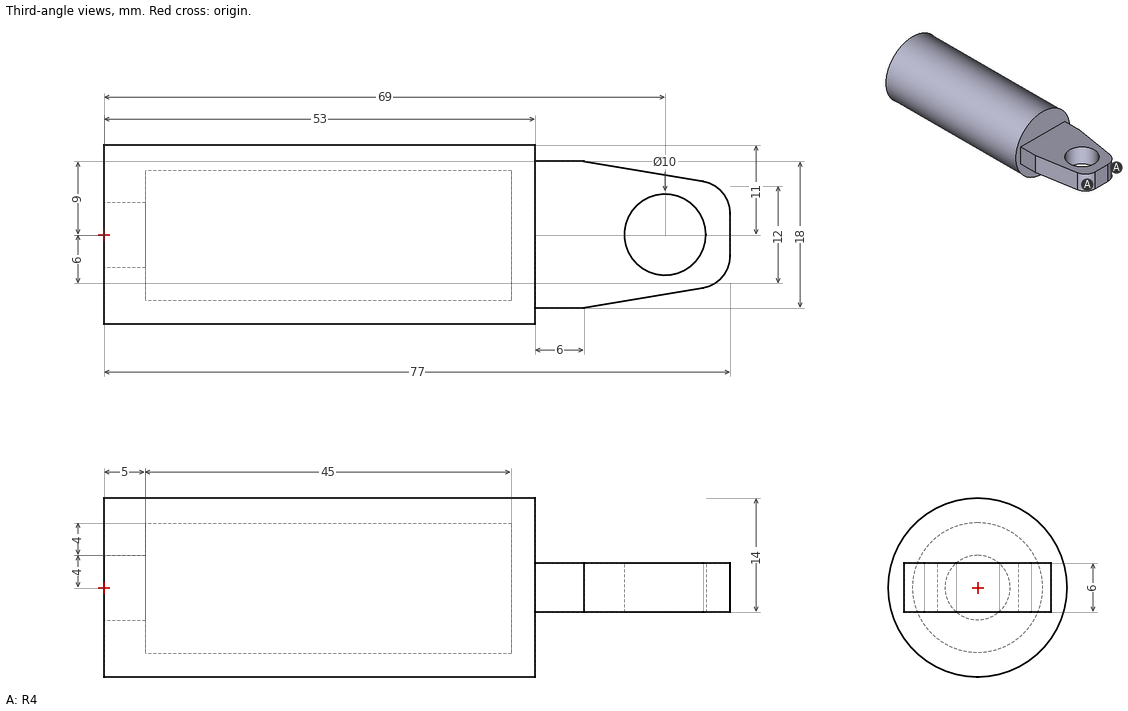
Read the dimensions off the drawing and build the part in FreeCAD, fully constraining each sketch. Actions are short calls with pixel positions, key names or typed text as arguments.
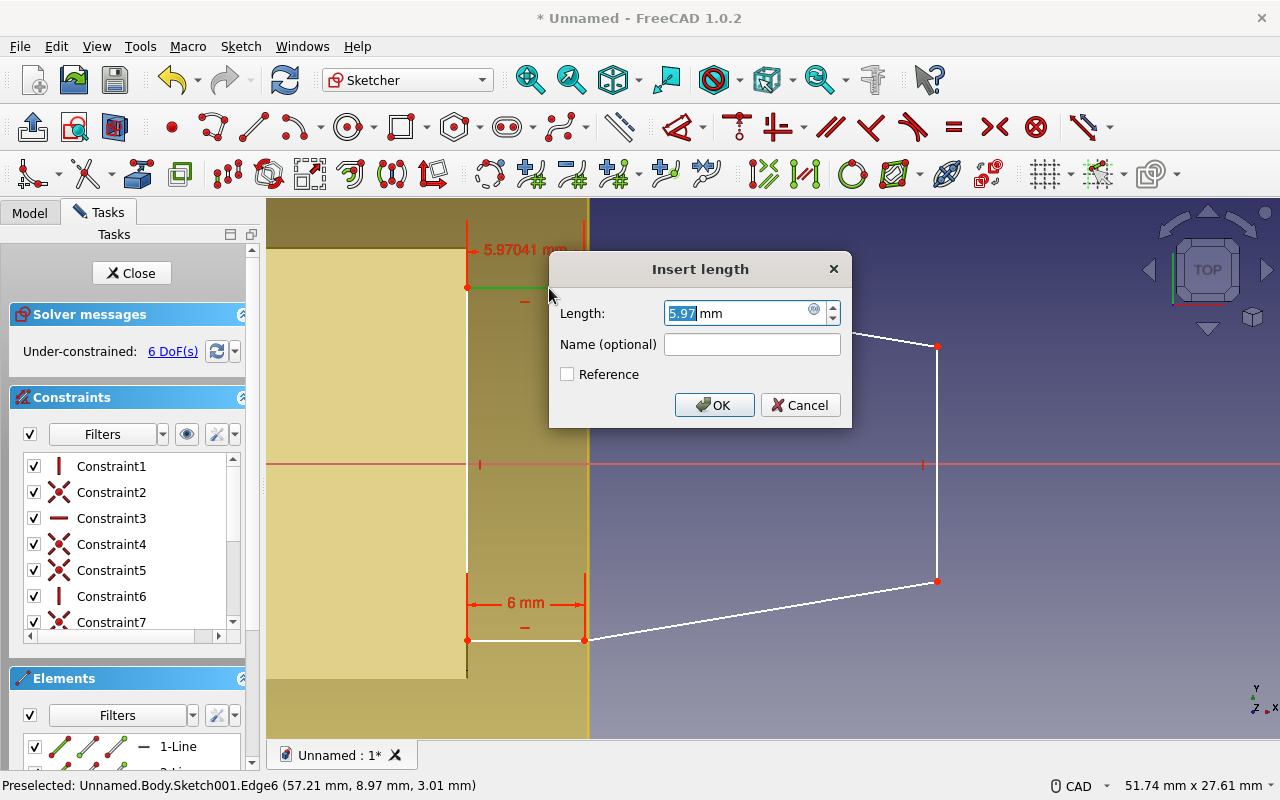
text(6)
key(Return)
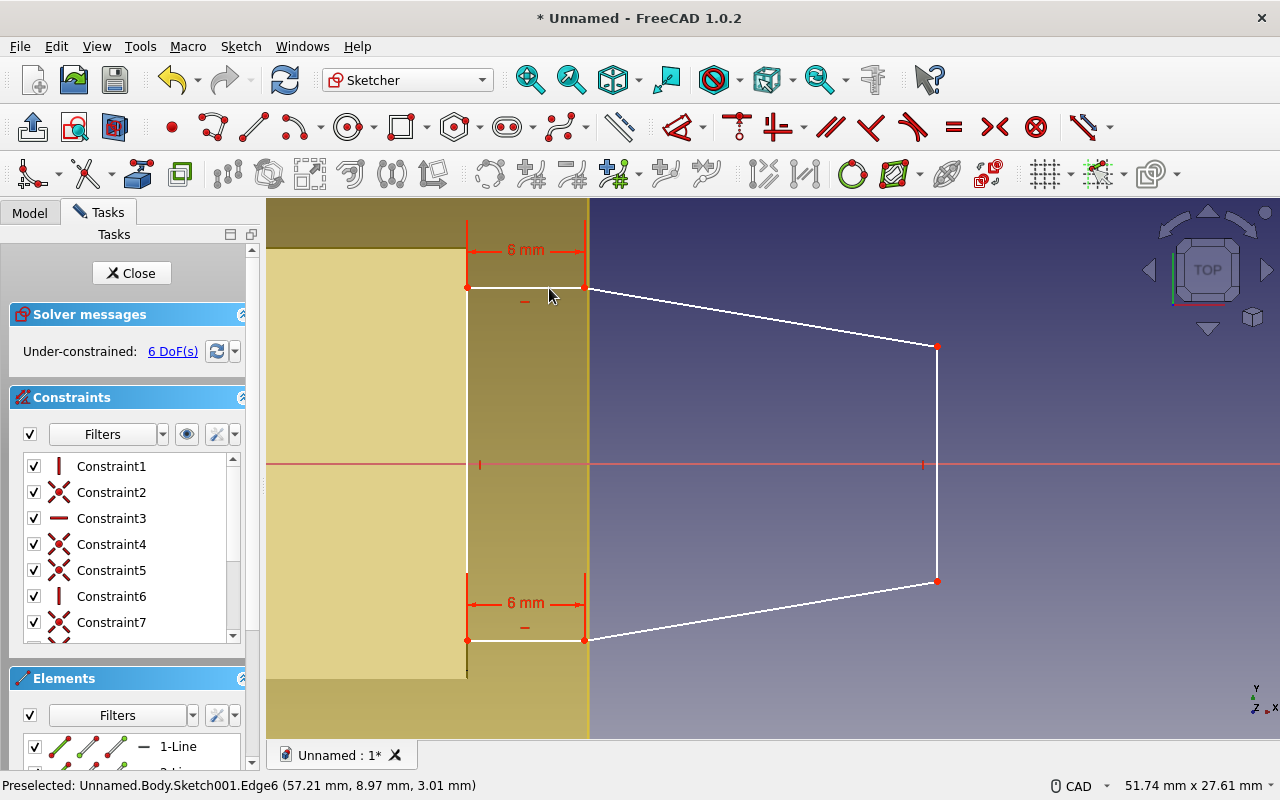
click(467, 394)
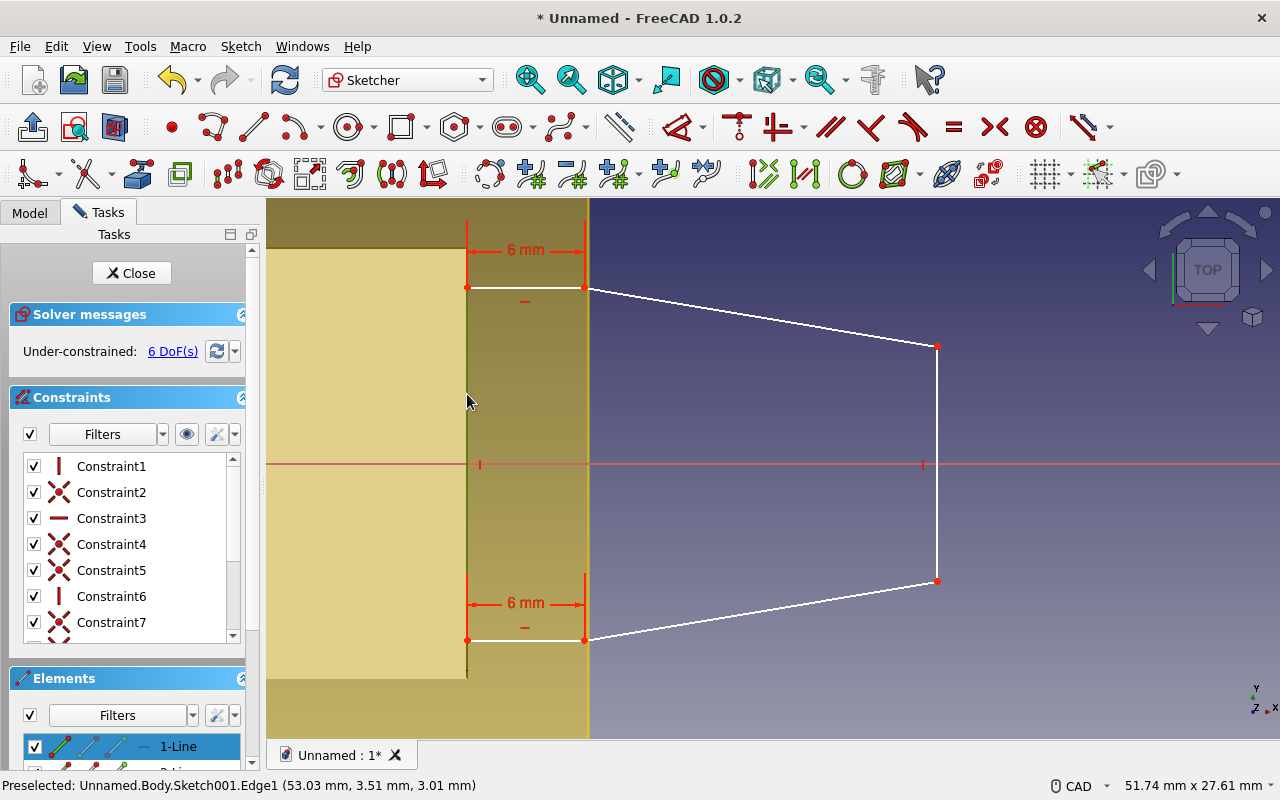
key(i)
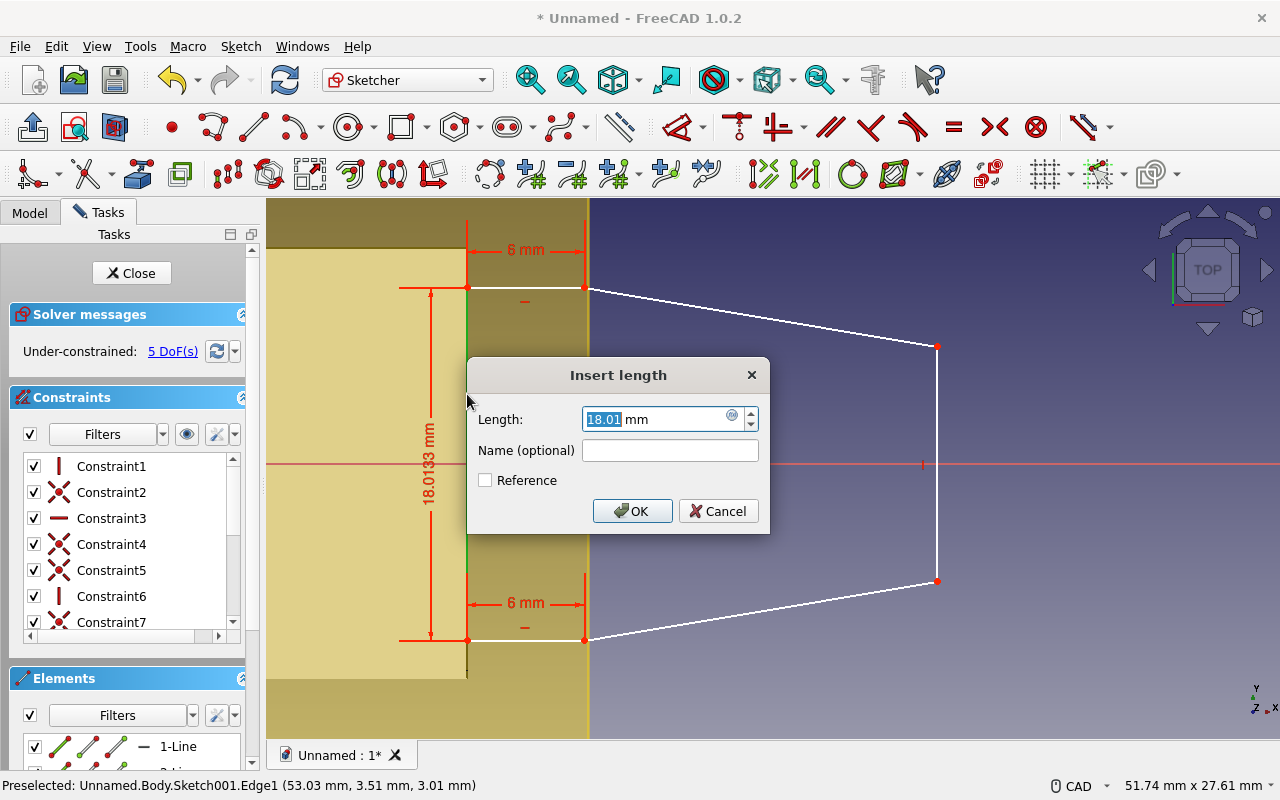
text(18)
key(Return)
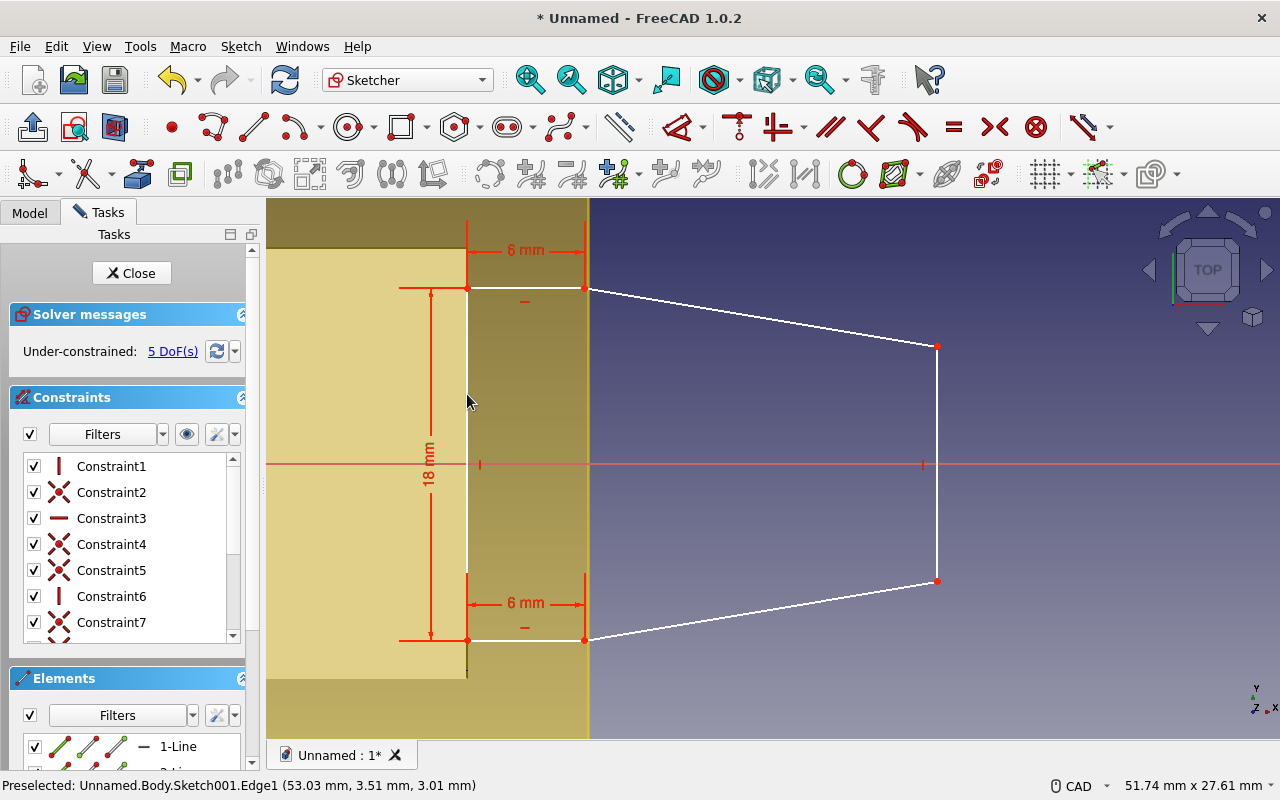
click(937, 511)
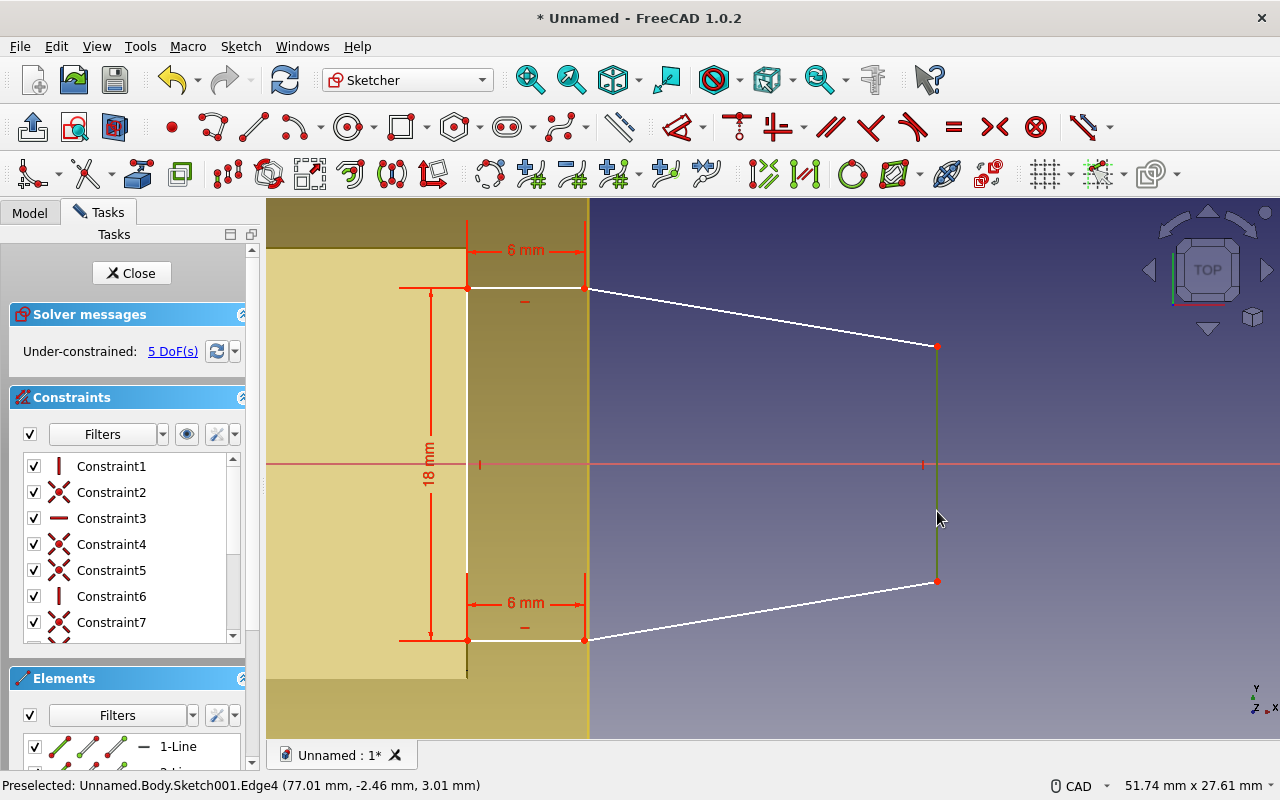
key(i)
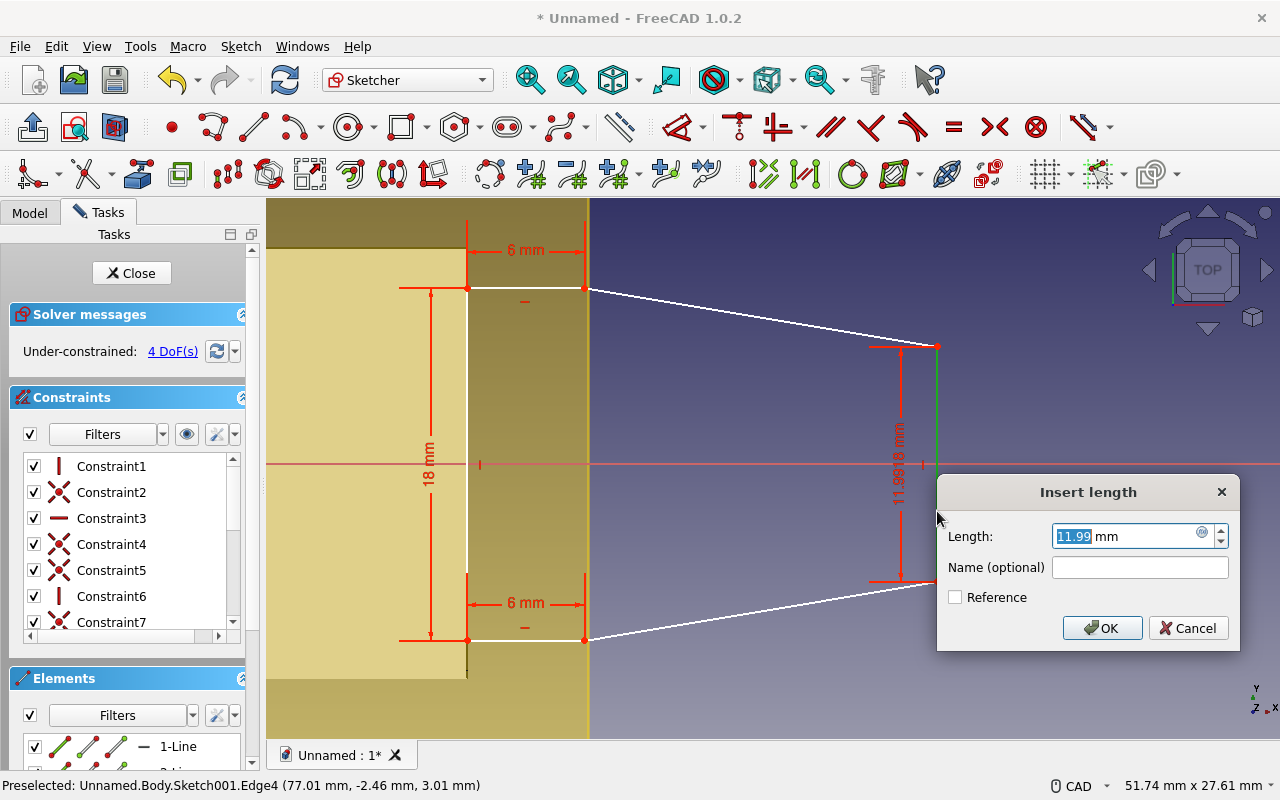
text(12)
key(Return)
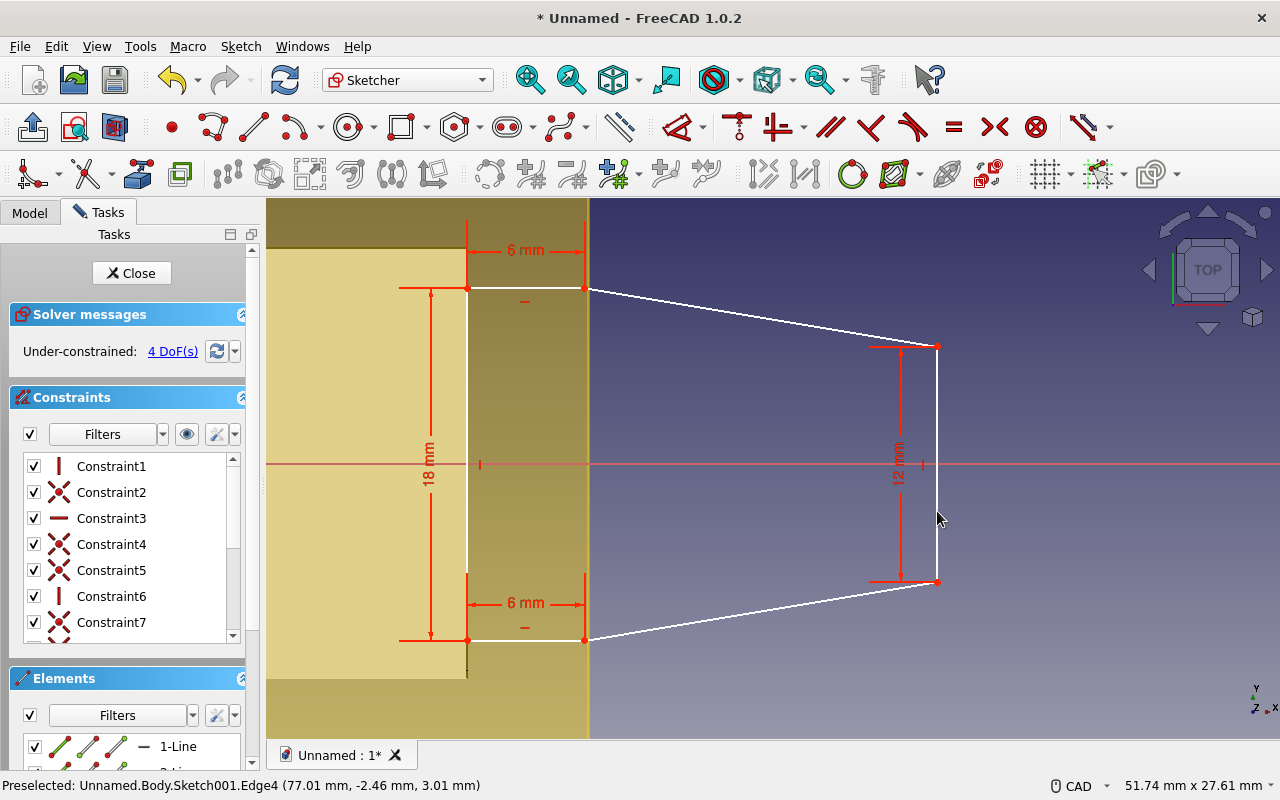
click(467, 288)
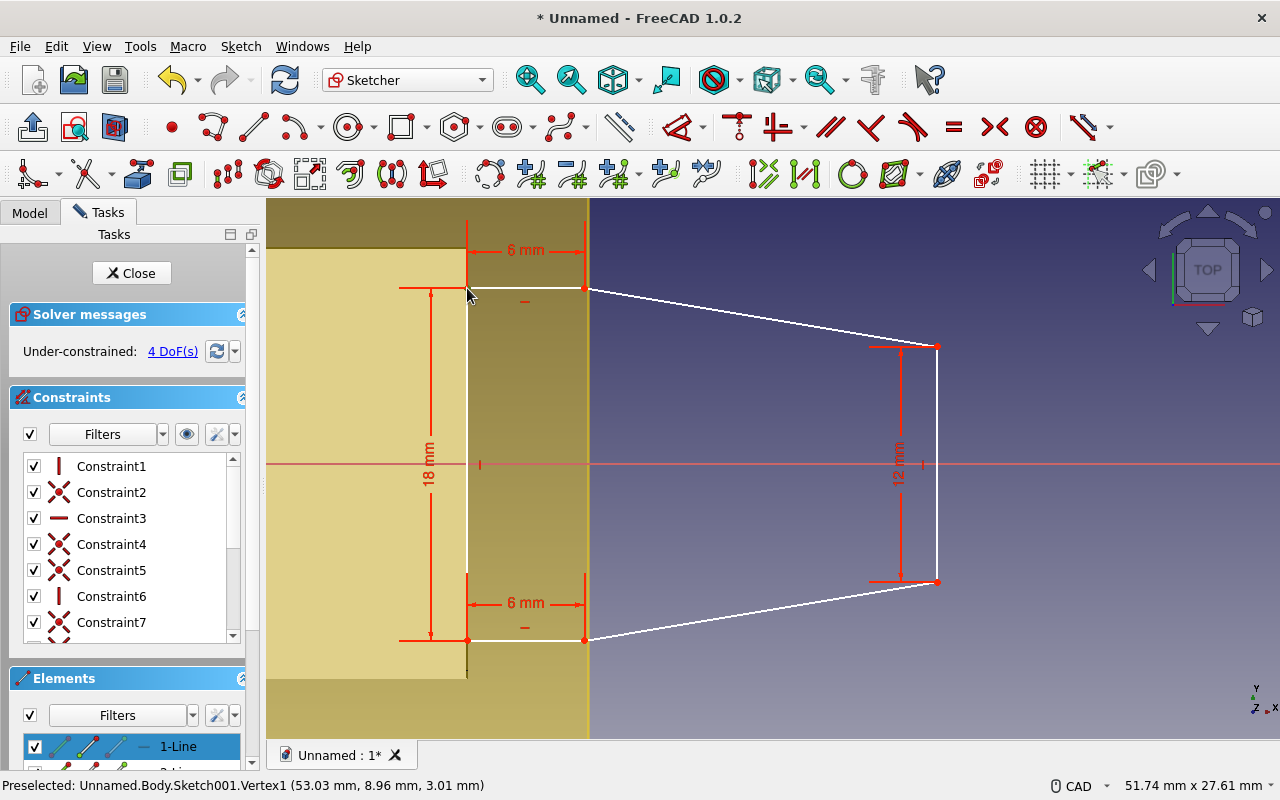
key(i)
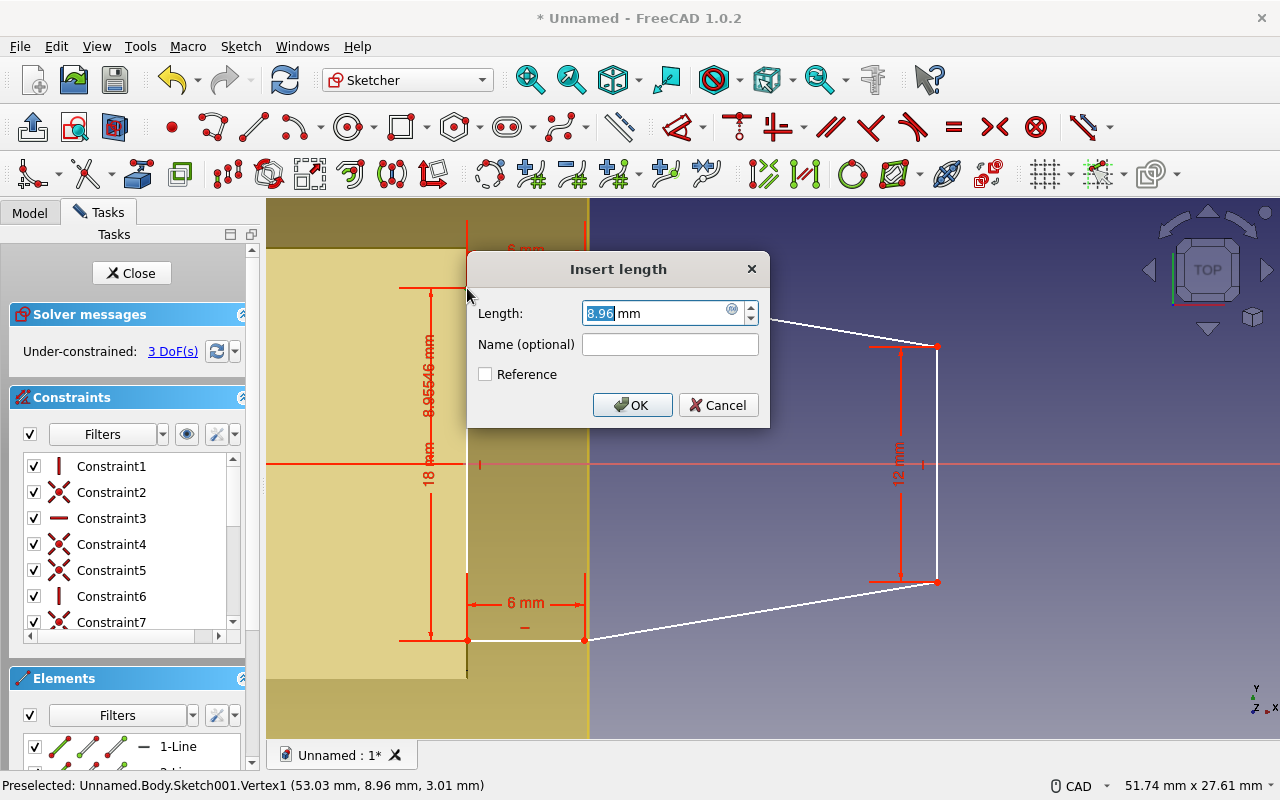
text(9)
key(Return)